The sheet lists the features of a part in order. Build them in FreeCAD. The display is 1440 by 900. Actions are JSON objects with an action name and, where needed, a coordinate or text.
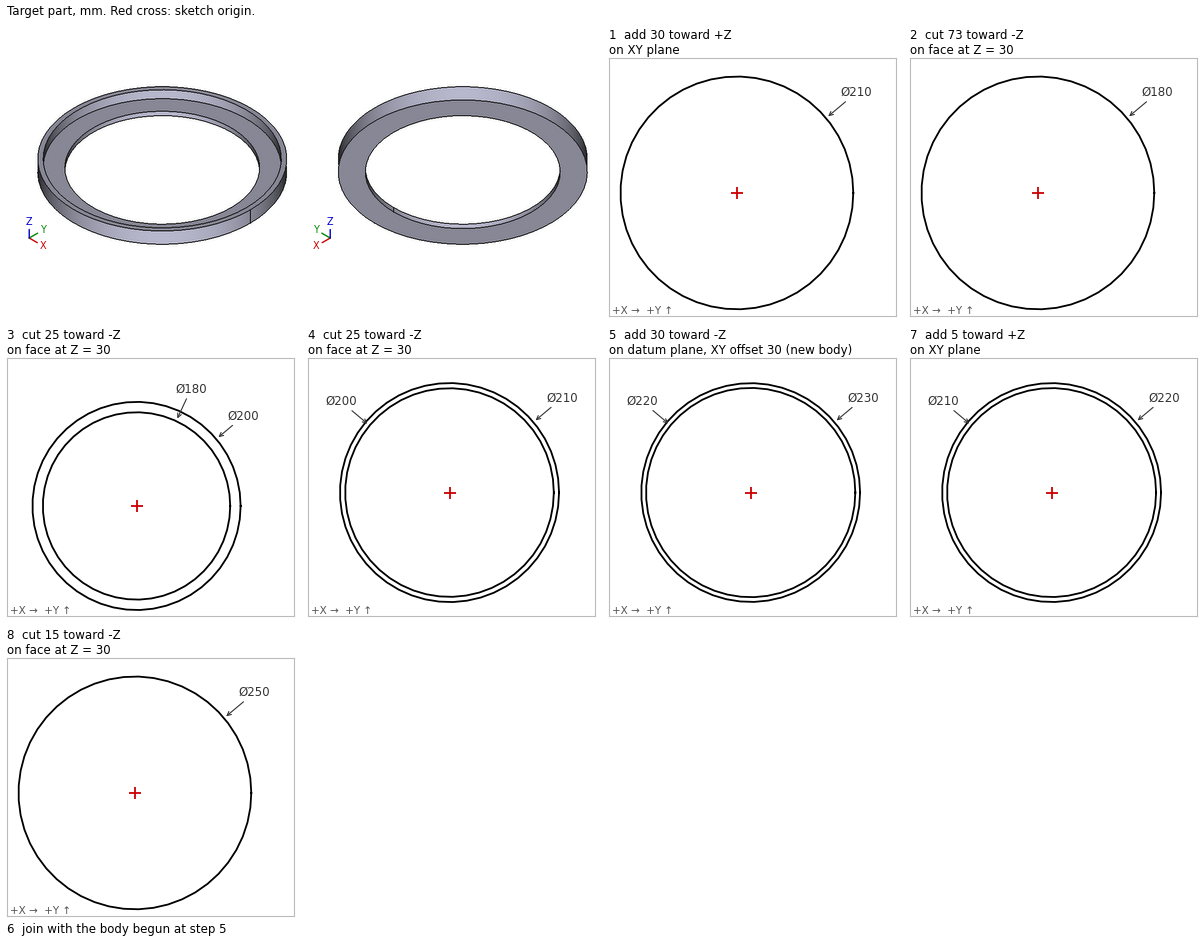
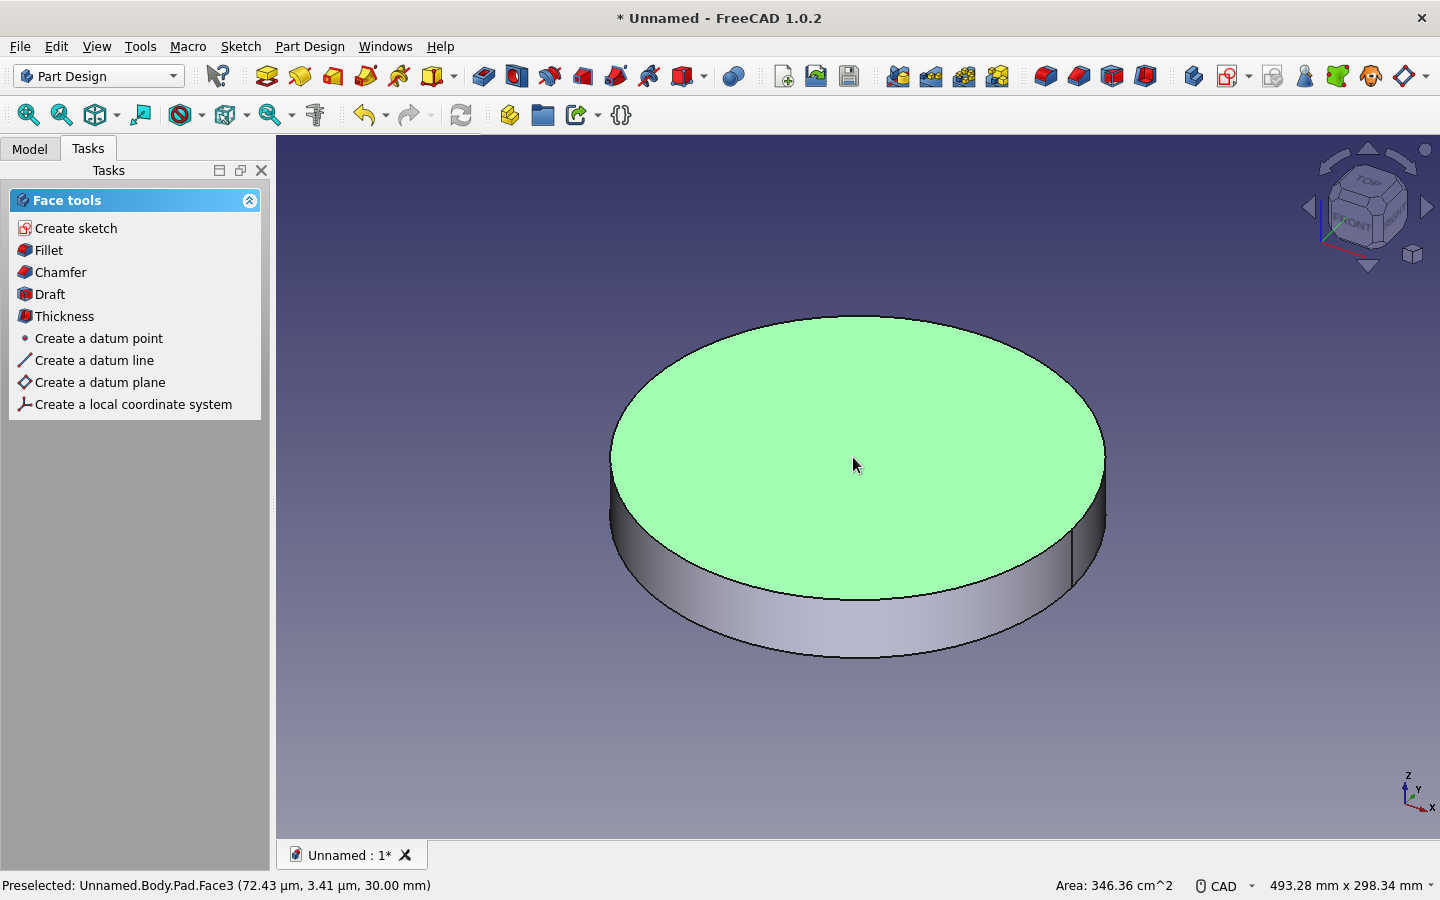
{"action": "left_click", "coordinate": [1226, 76]}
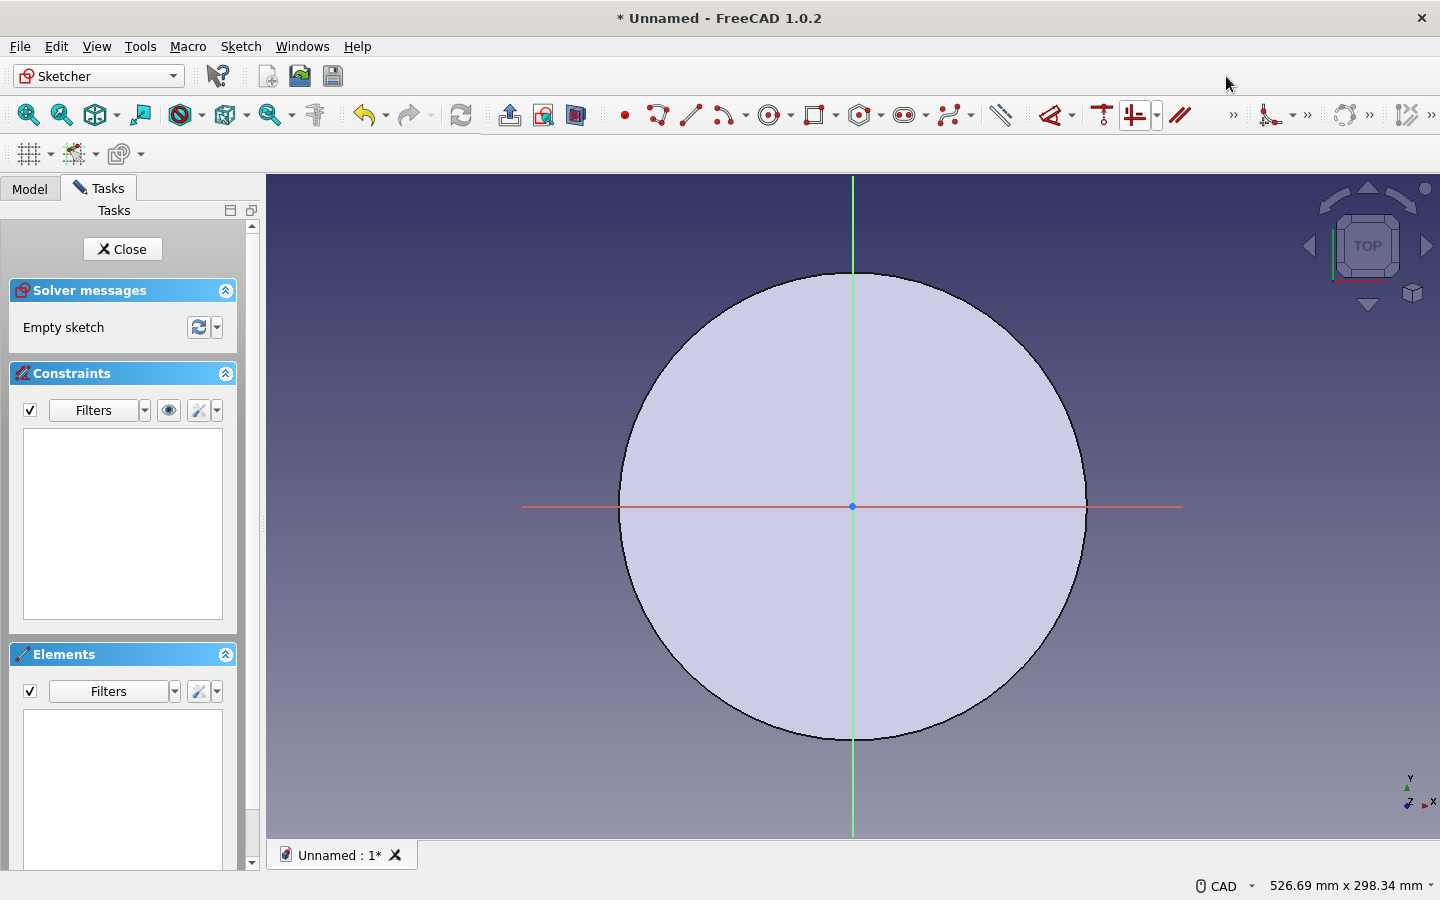
{"action": "left_click", "coordinate": [768, 116]}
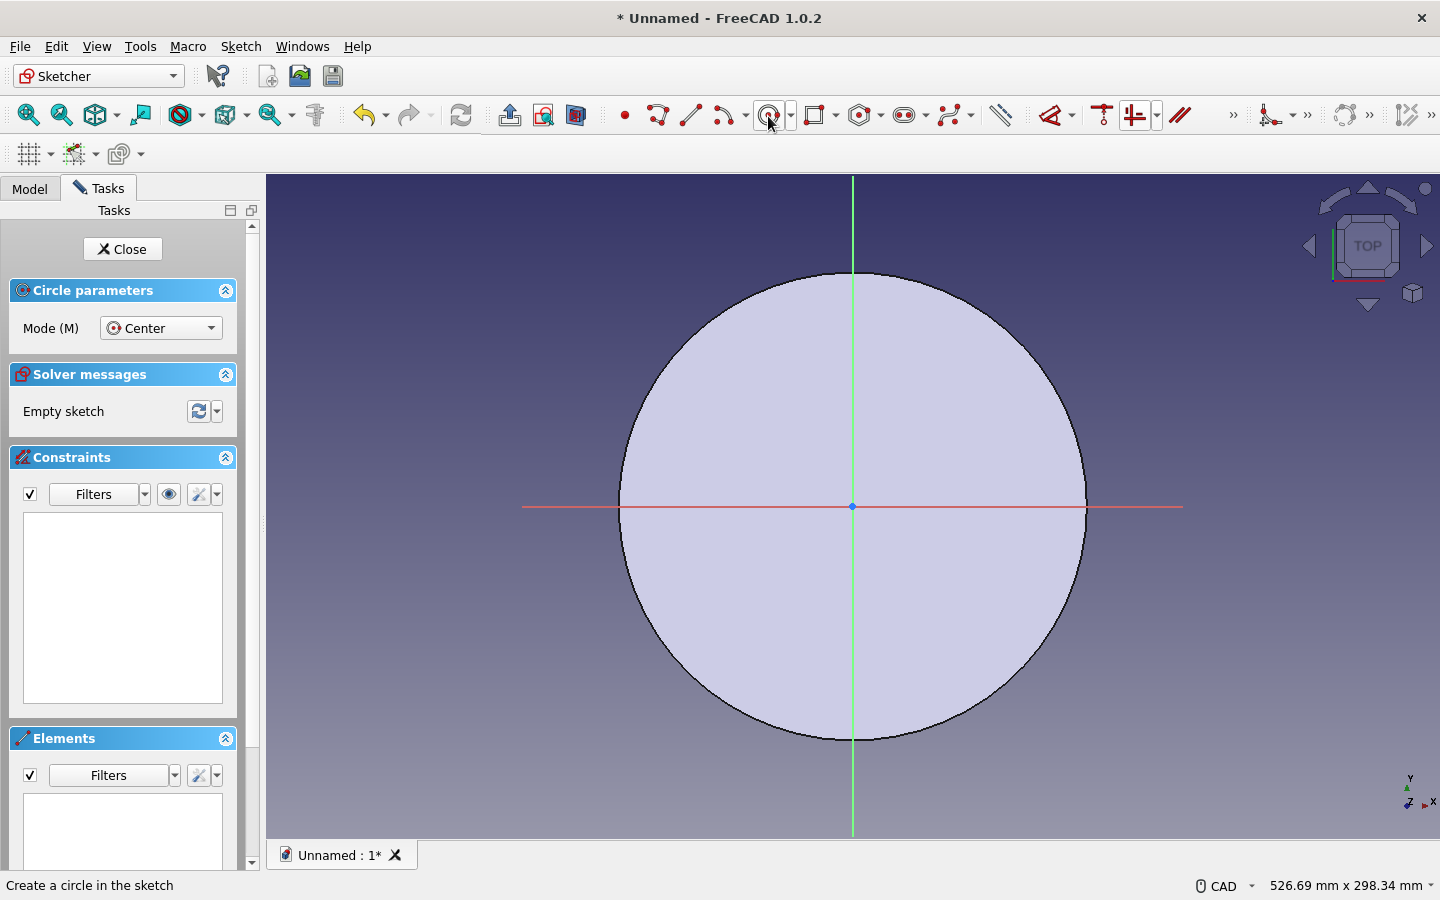
{"action": "left_click", "coordinate": [853, 506]}
{"action": "mouse_move", "coordinate": [995, 365]}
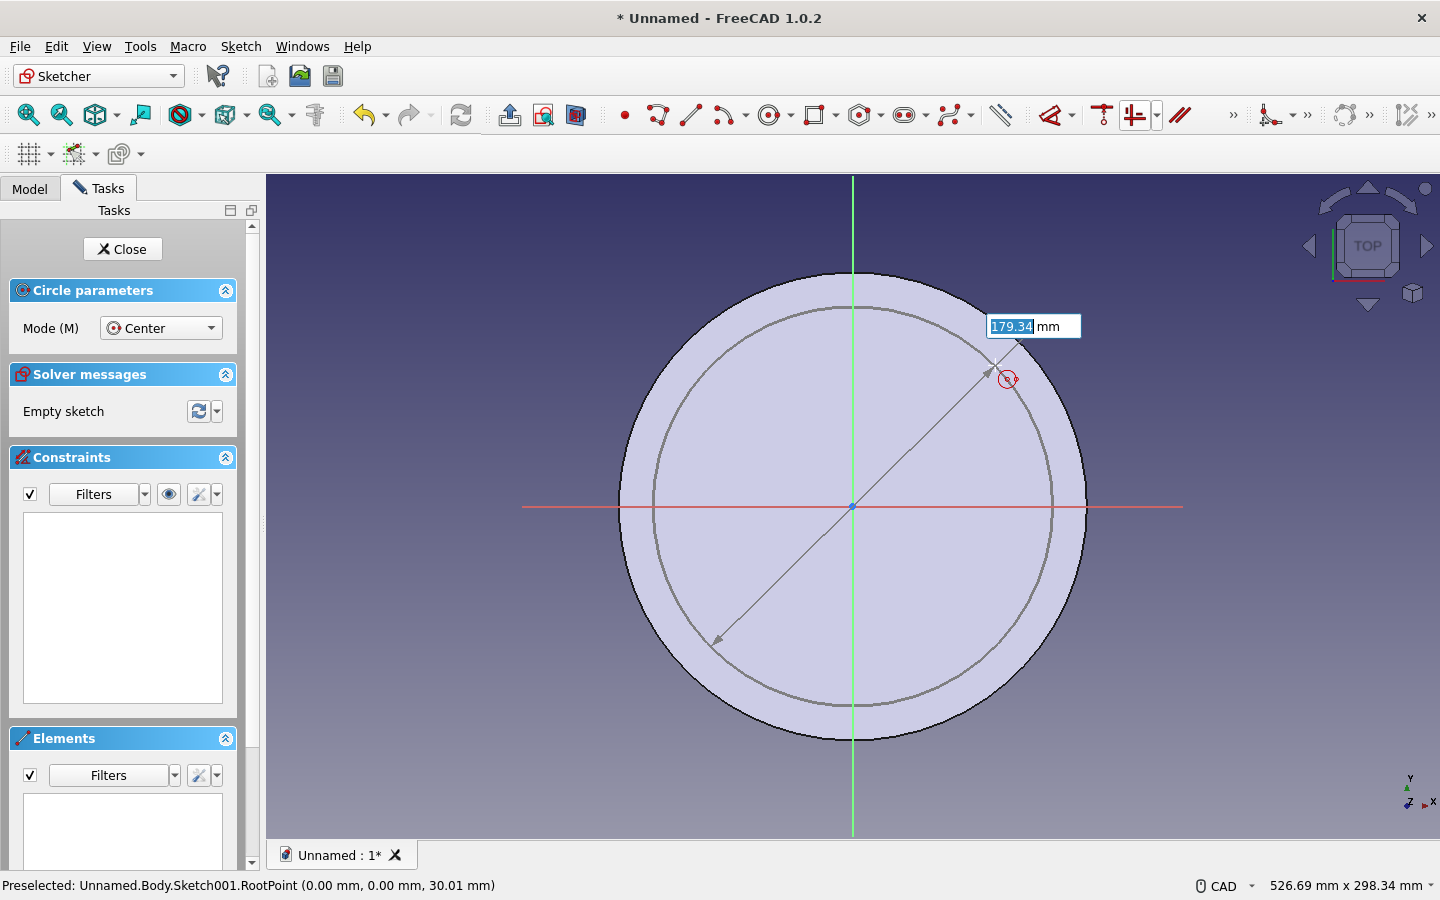
{"action": "type", "text": "180"}
{"action": "key", "text": "Return"}
{"action": "key", "text": "Escape"}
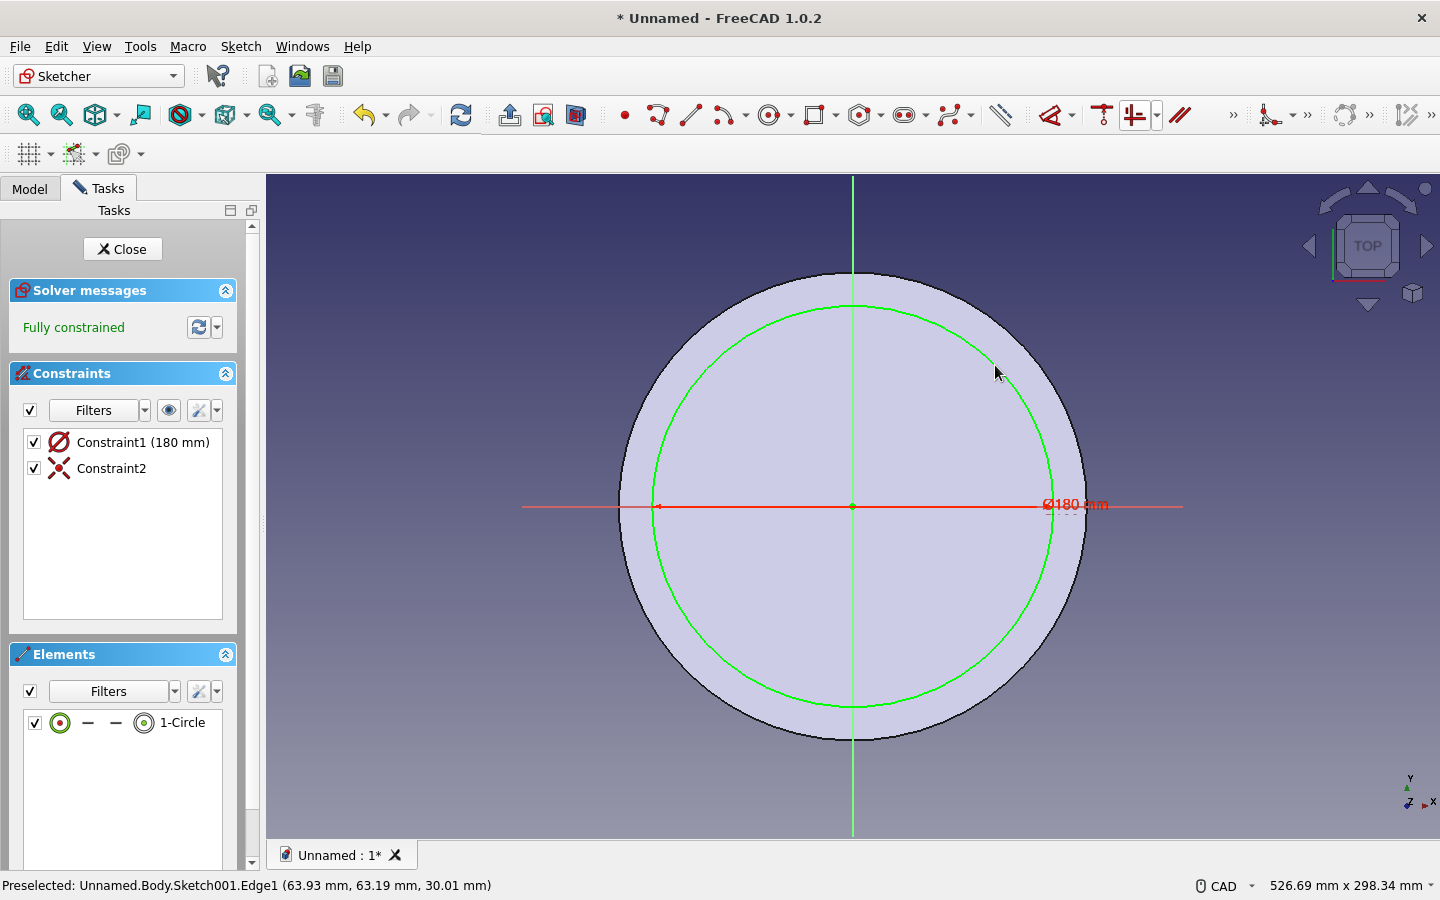
{"action": "left_click", "coordinate": [123, 249]}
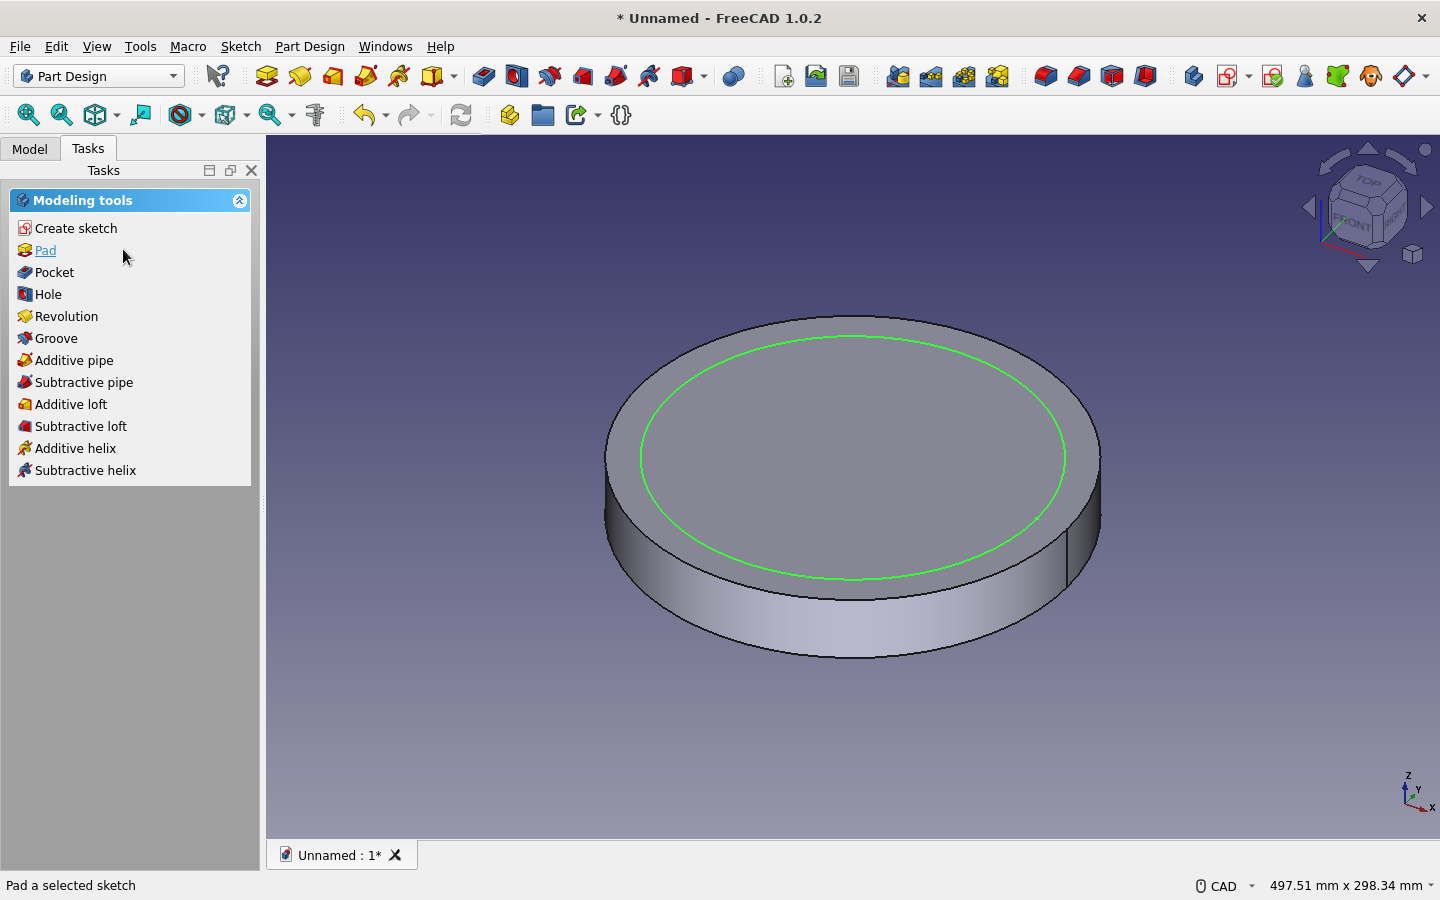
{"action": "left_click", "coordinate": [484, 76]}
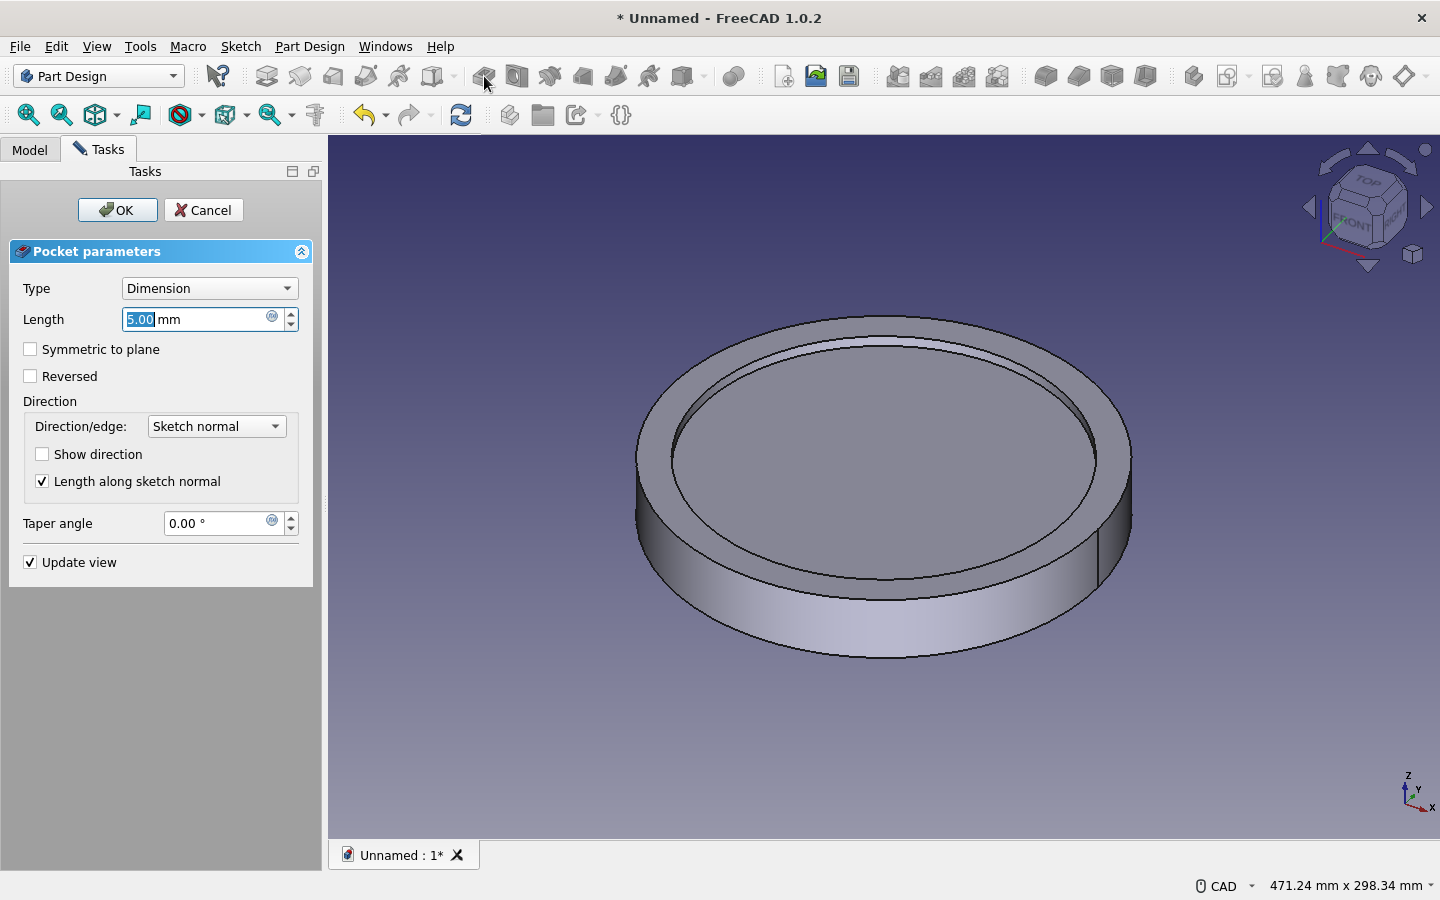
{"action": "type", "text": "73"}
{"action": "key", "text": "Tab"}